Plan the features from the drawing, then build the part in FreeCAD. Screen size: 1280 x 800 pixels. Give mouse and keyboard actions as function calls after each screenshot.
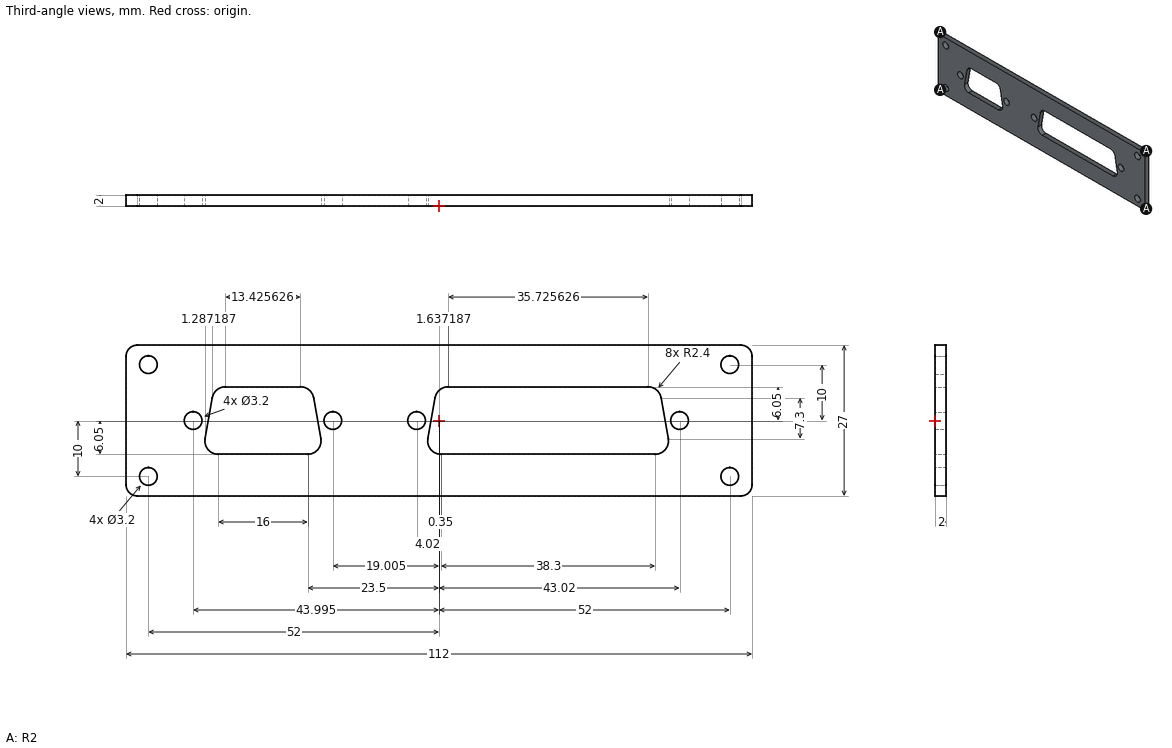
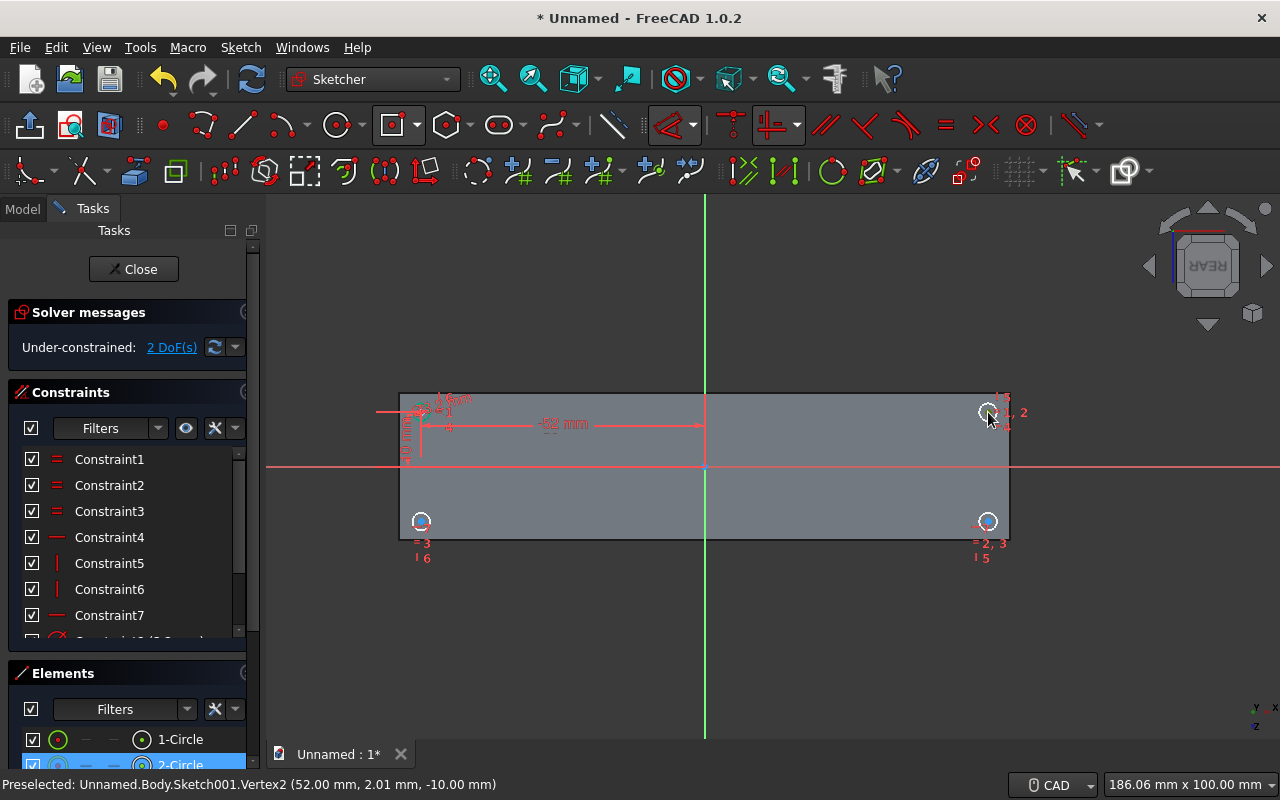
click(696, 126)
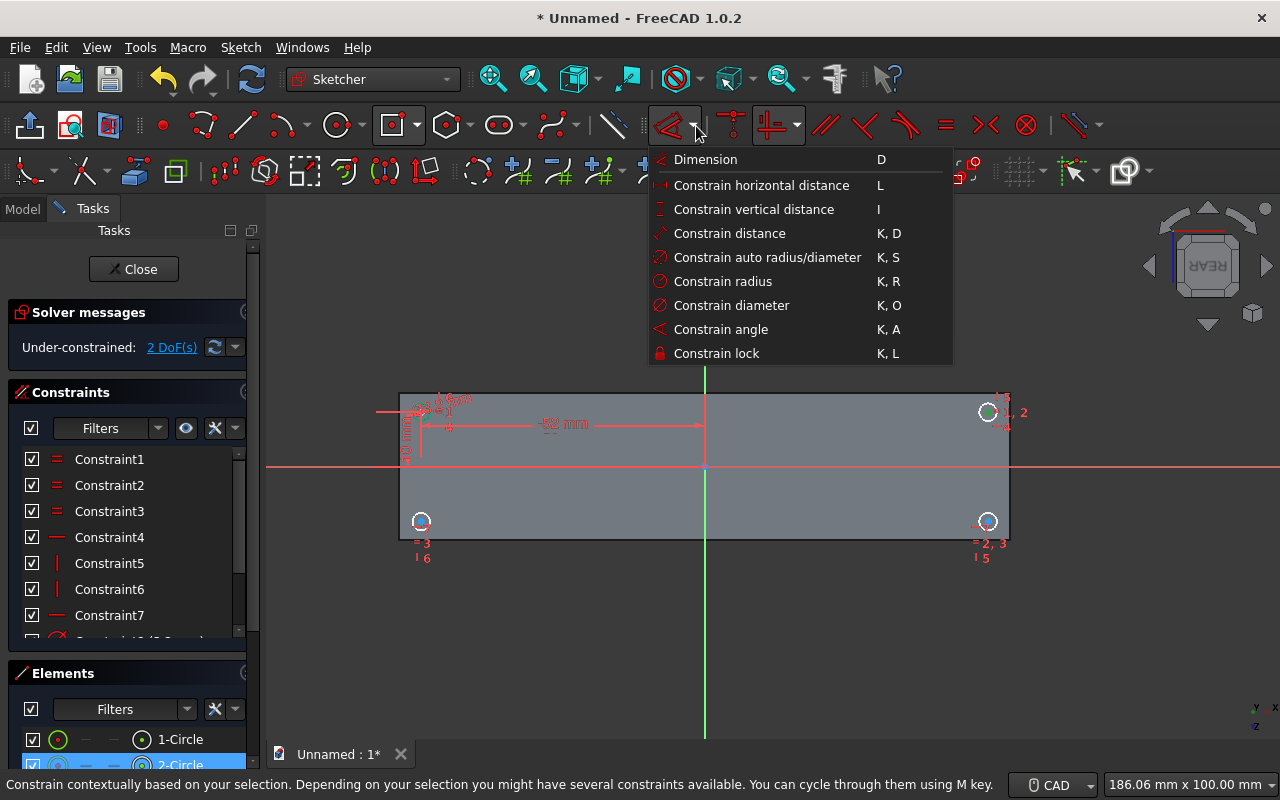
click(801, 185)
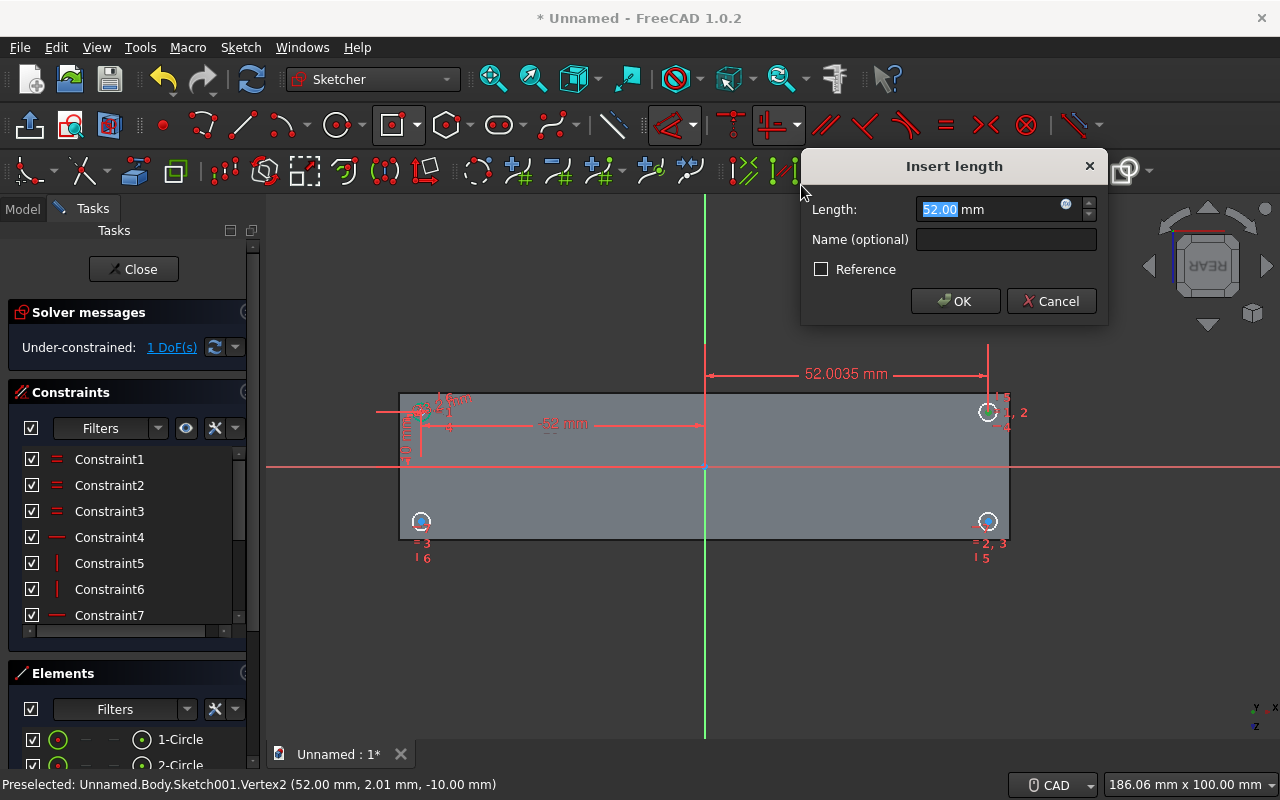
text(52)
key(Return)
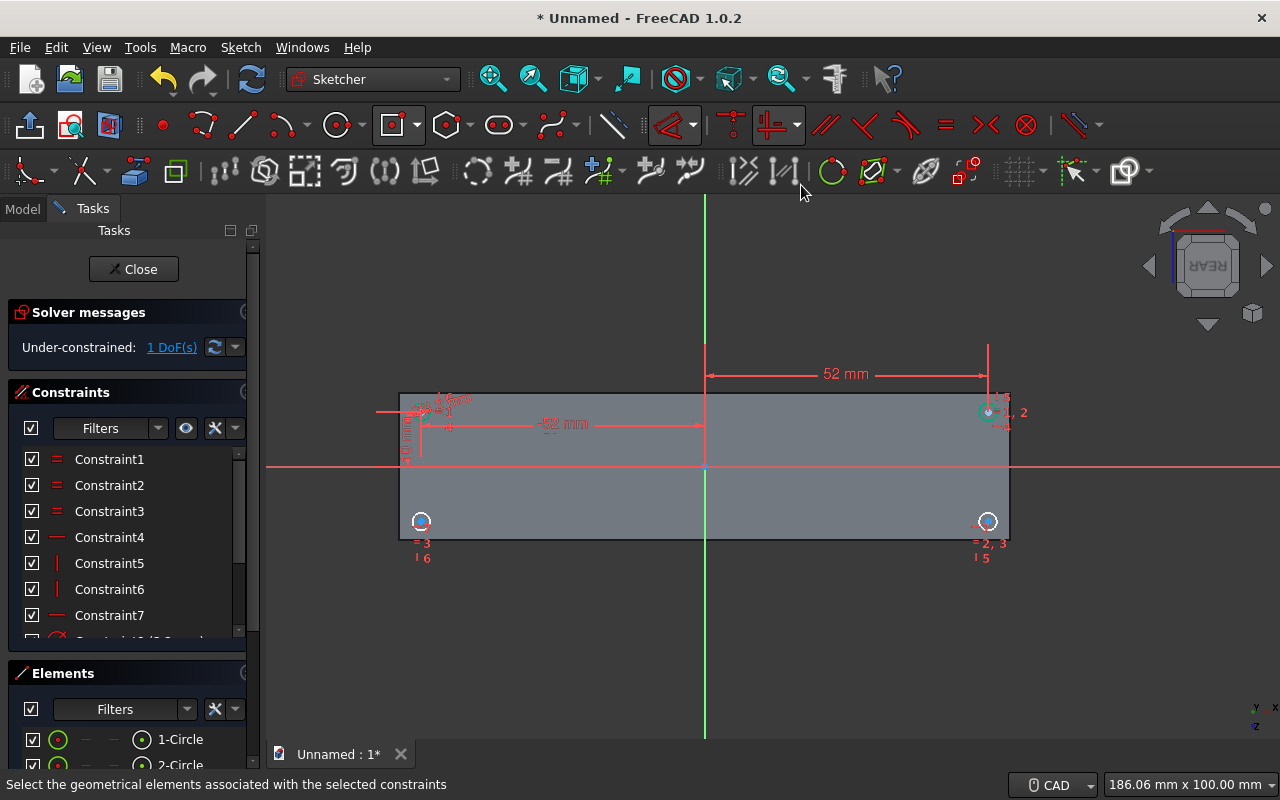
click(988, 522)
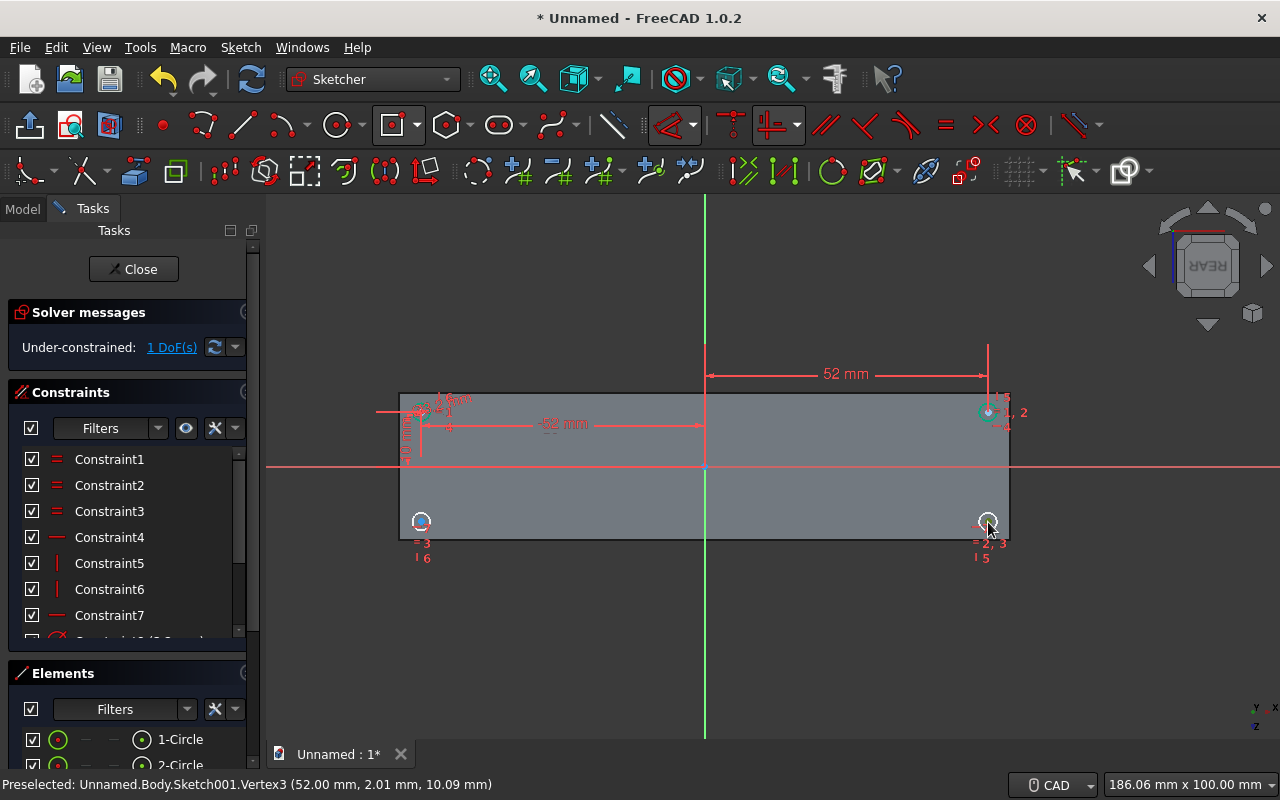
click(696, 126)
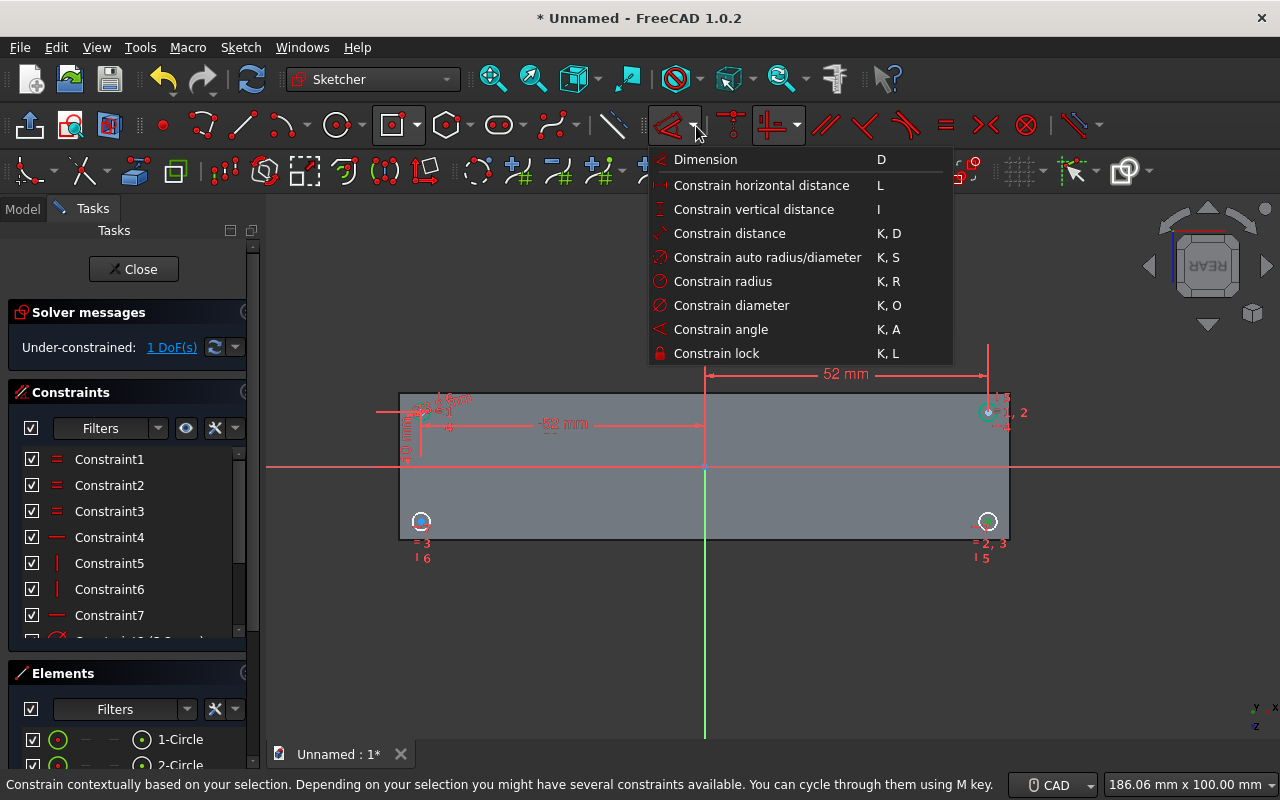
click(801, 209)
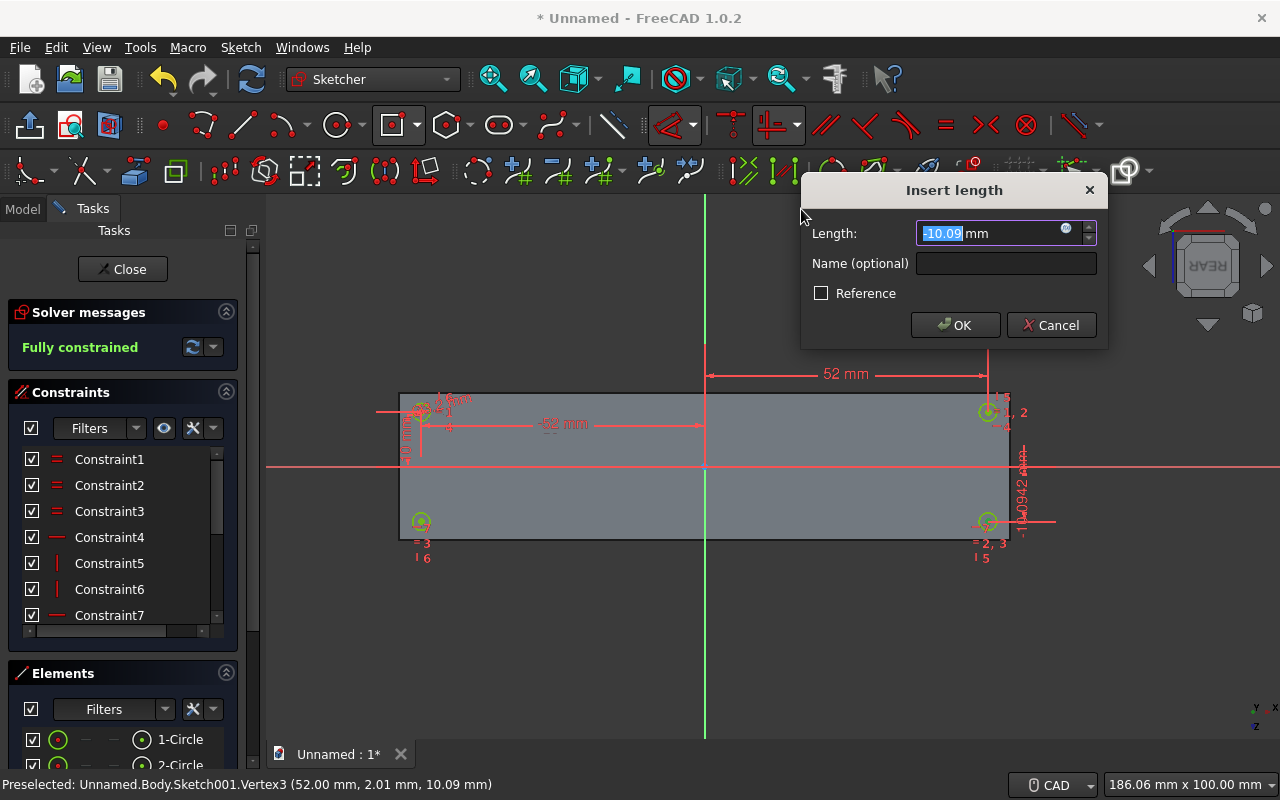
text(-10)
key(Return)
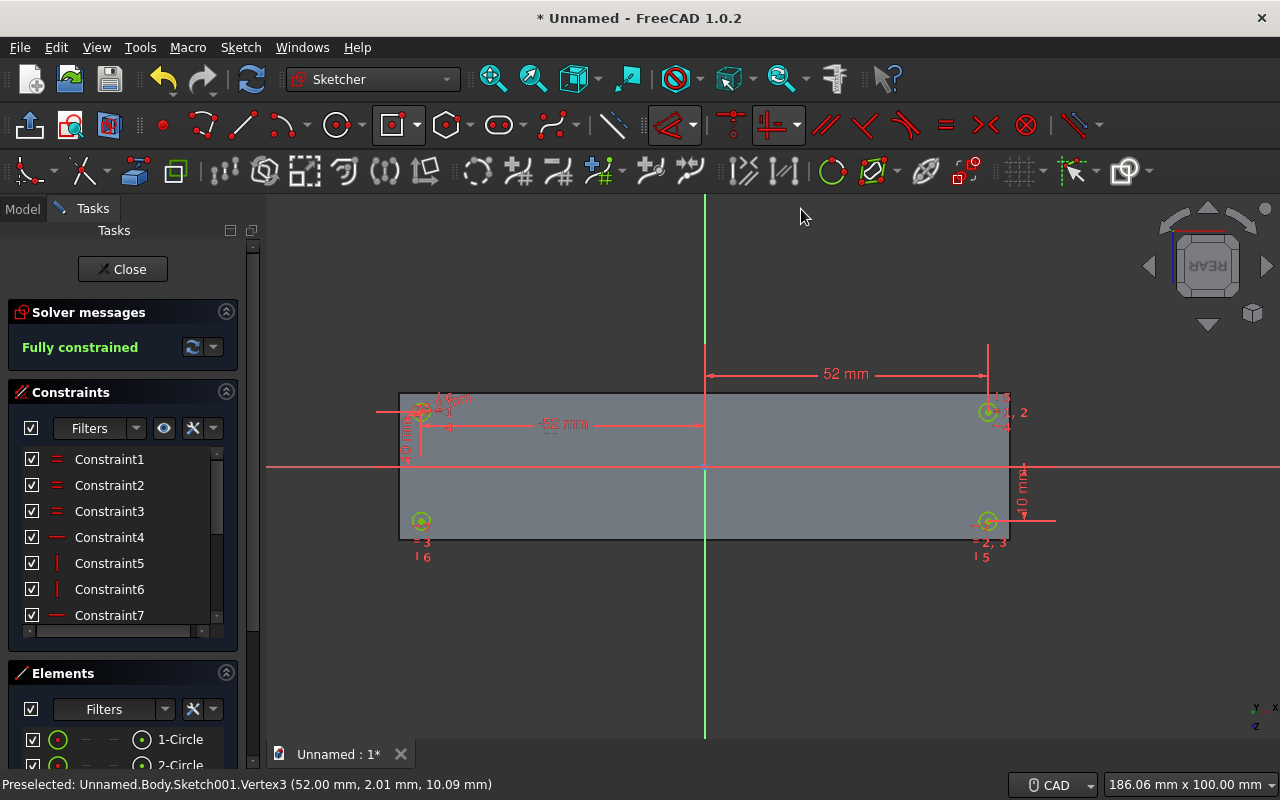
click(123, 269)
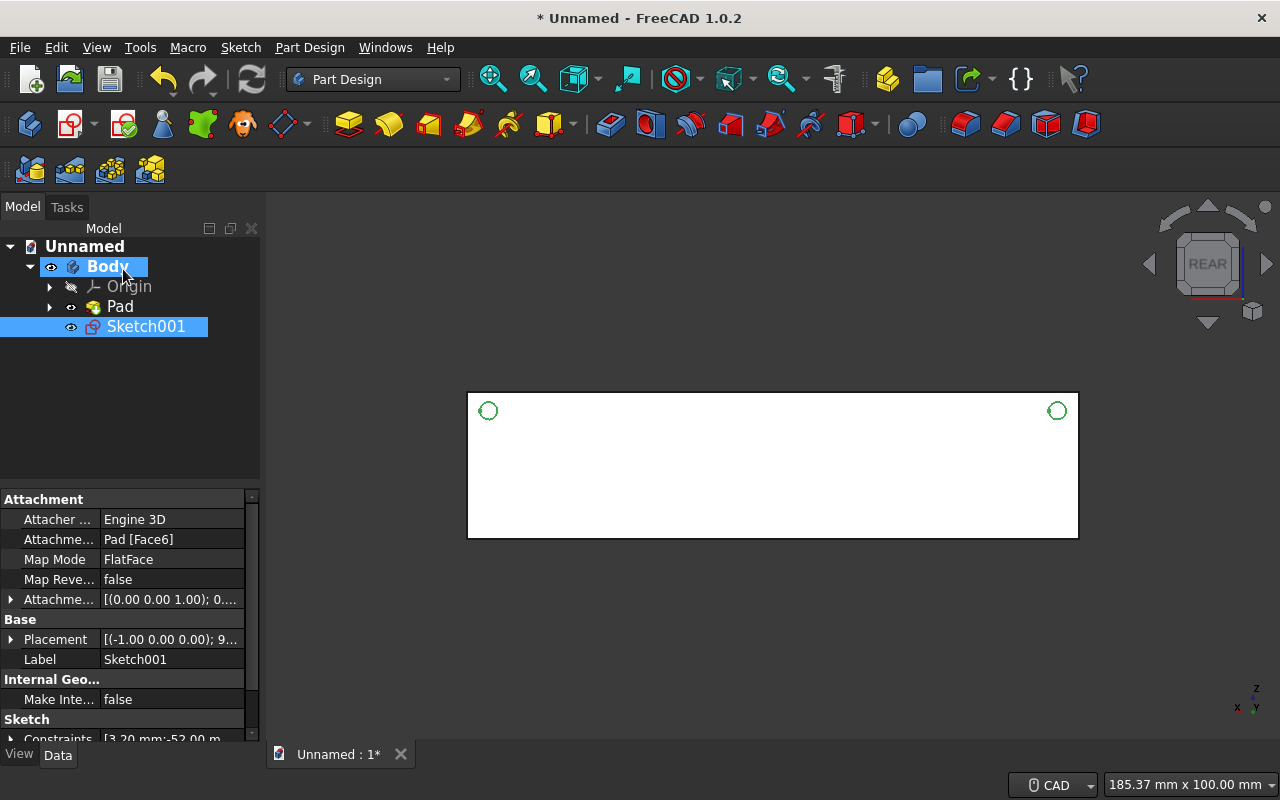
click(612, 124)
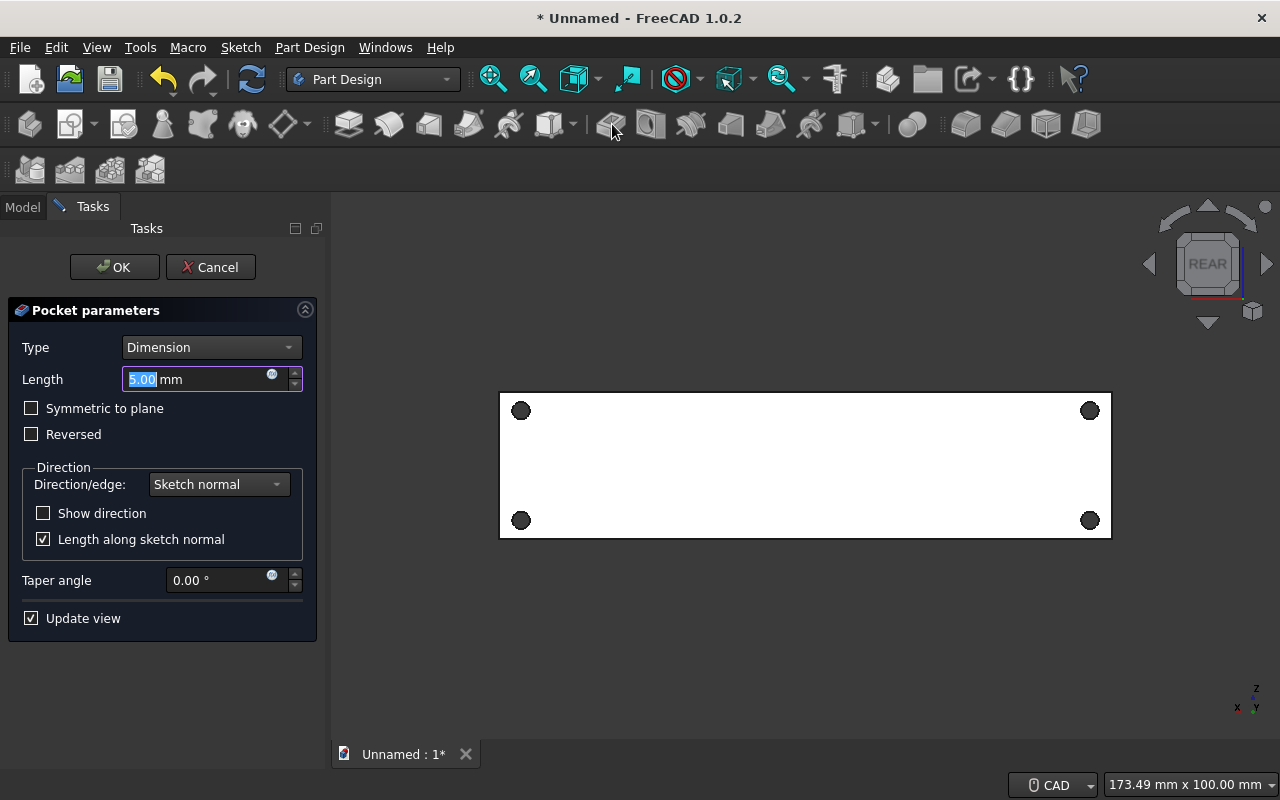
click(212, 348)